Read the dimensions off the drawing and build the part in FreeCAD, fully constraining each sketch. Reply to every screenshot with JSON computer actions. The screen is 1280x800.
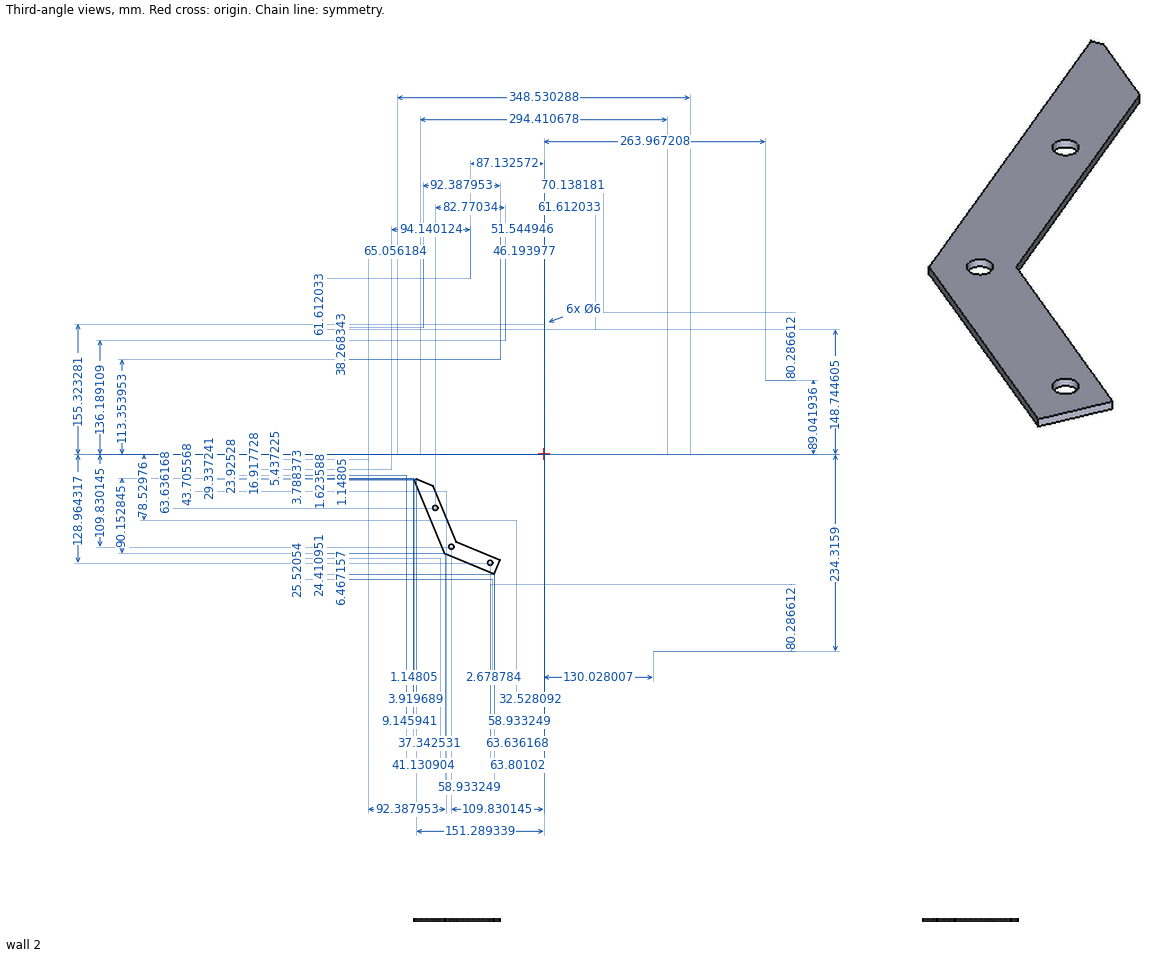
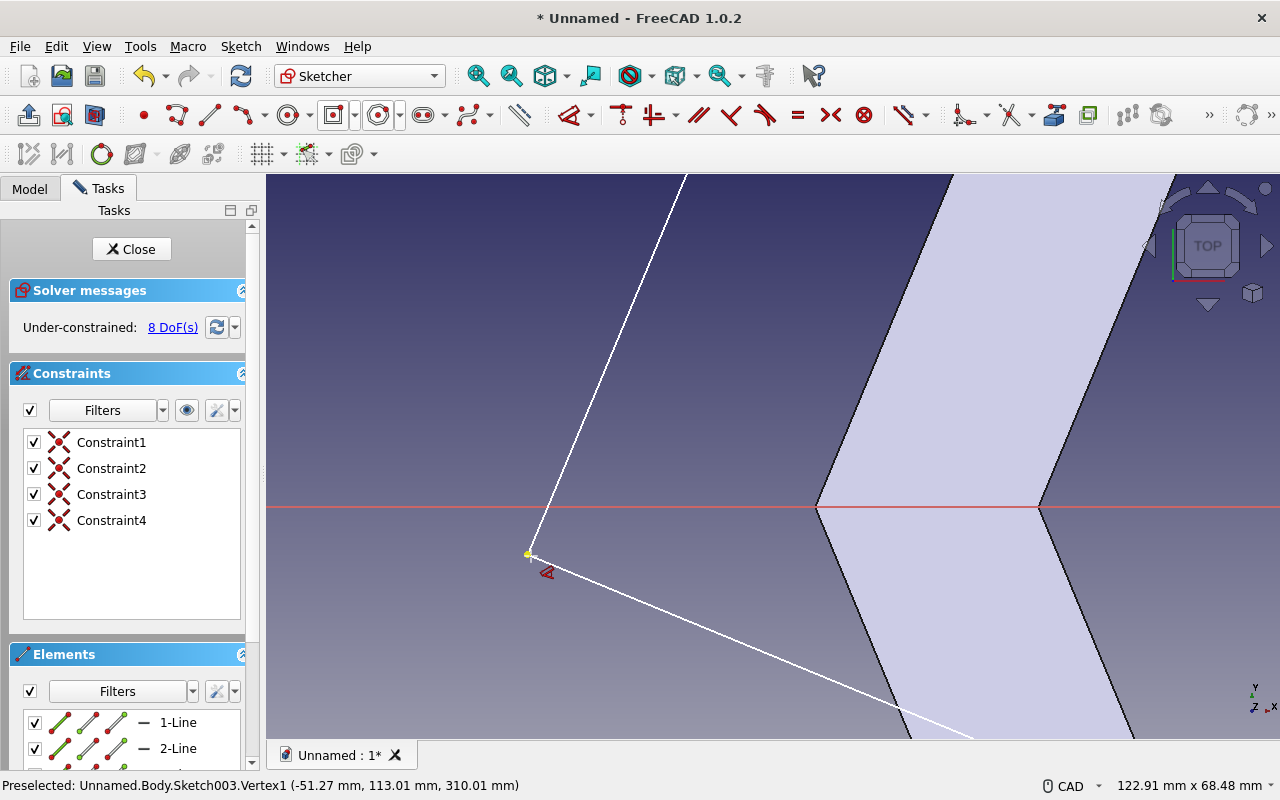
{"action": "left_click", "coordinate": [528, 555]}
{"action": "left_click", "coordinate": [494, 531]}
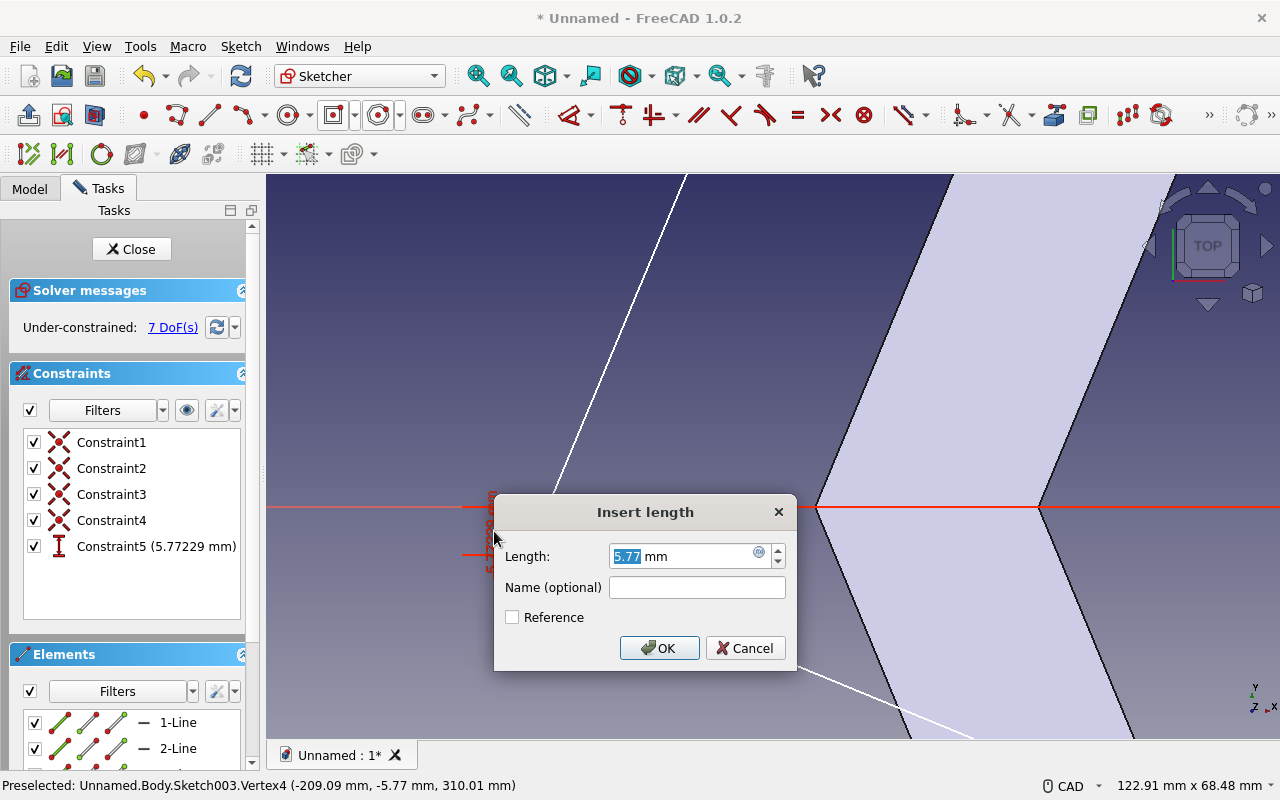
{"action": "type", "text": "5.437225"}
{"action": "key", "text": "Return"}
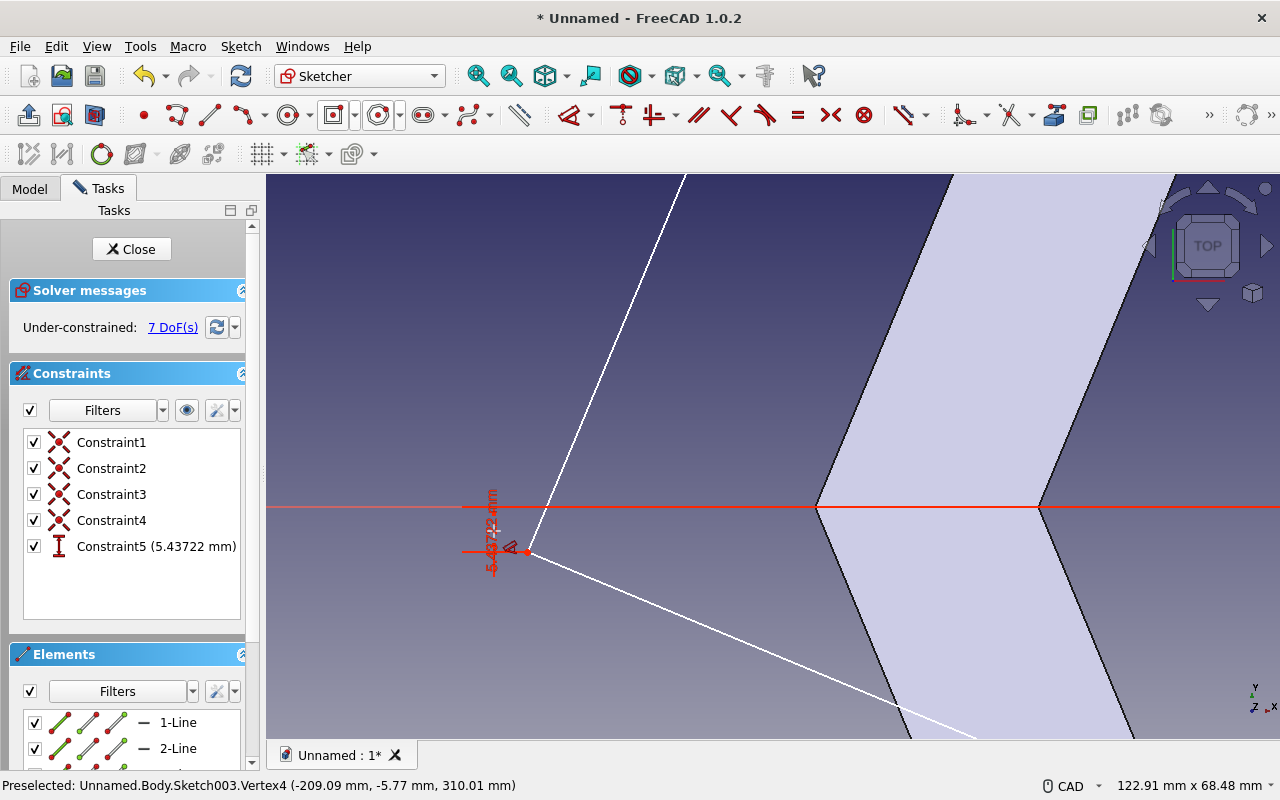
{"action": "scroll", "coordinate": [531, 556], "scroll_direction": "down", "scroll_amount": 8}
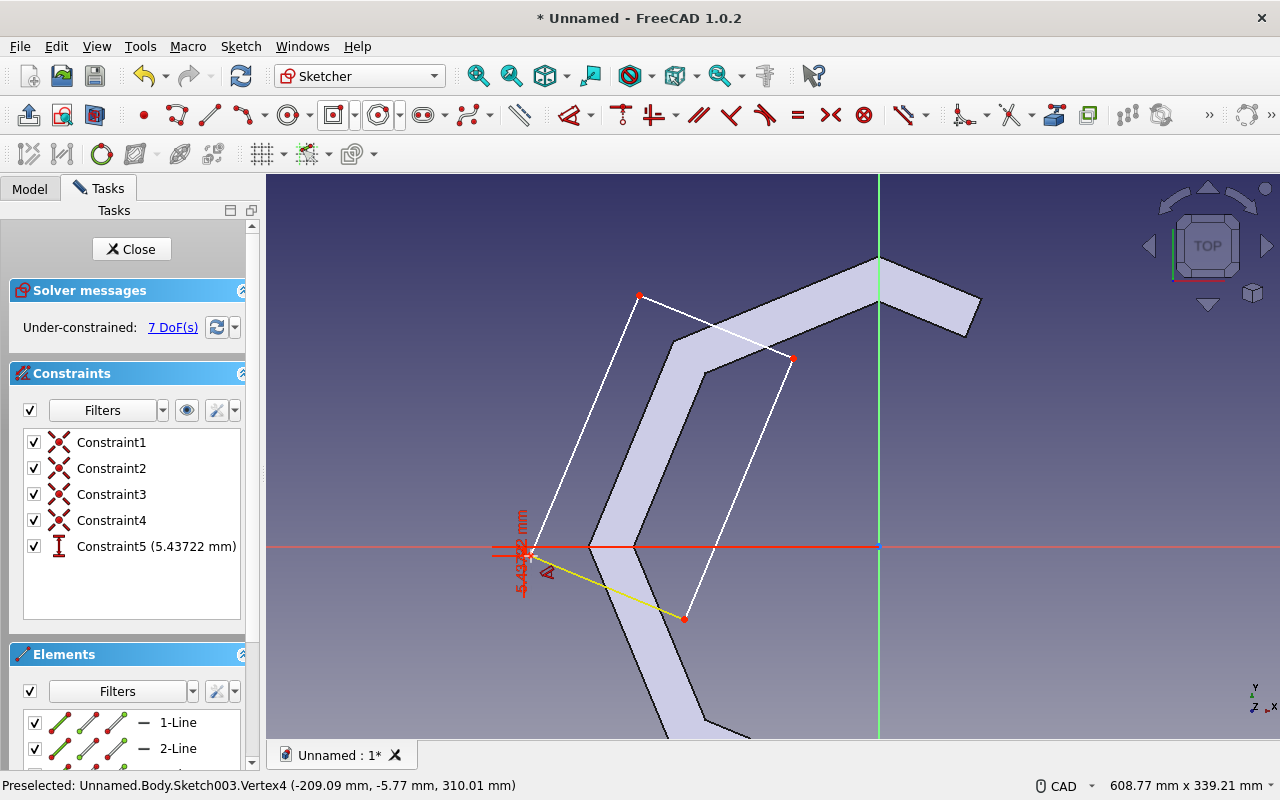
{"action": "left_click", "coordinate": [793, 358]}
{"action": "left_click", "coordinate": [836, 324]}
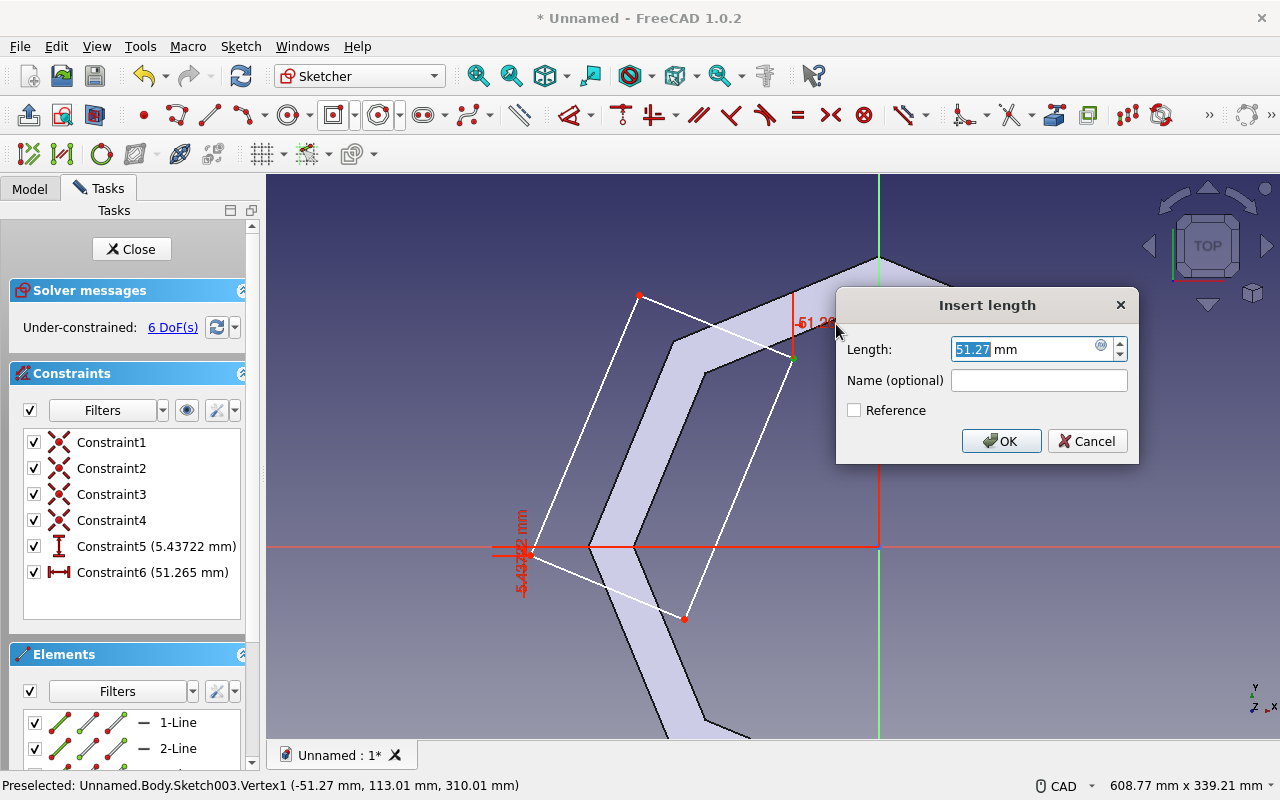
{"action": "type", "text": "51.544946"}
{"action": "key", "text": "Return"}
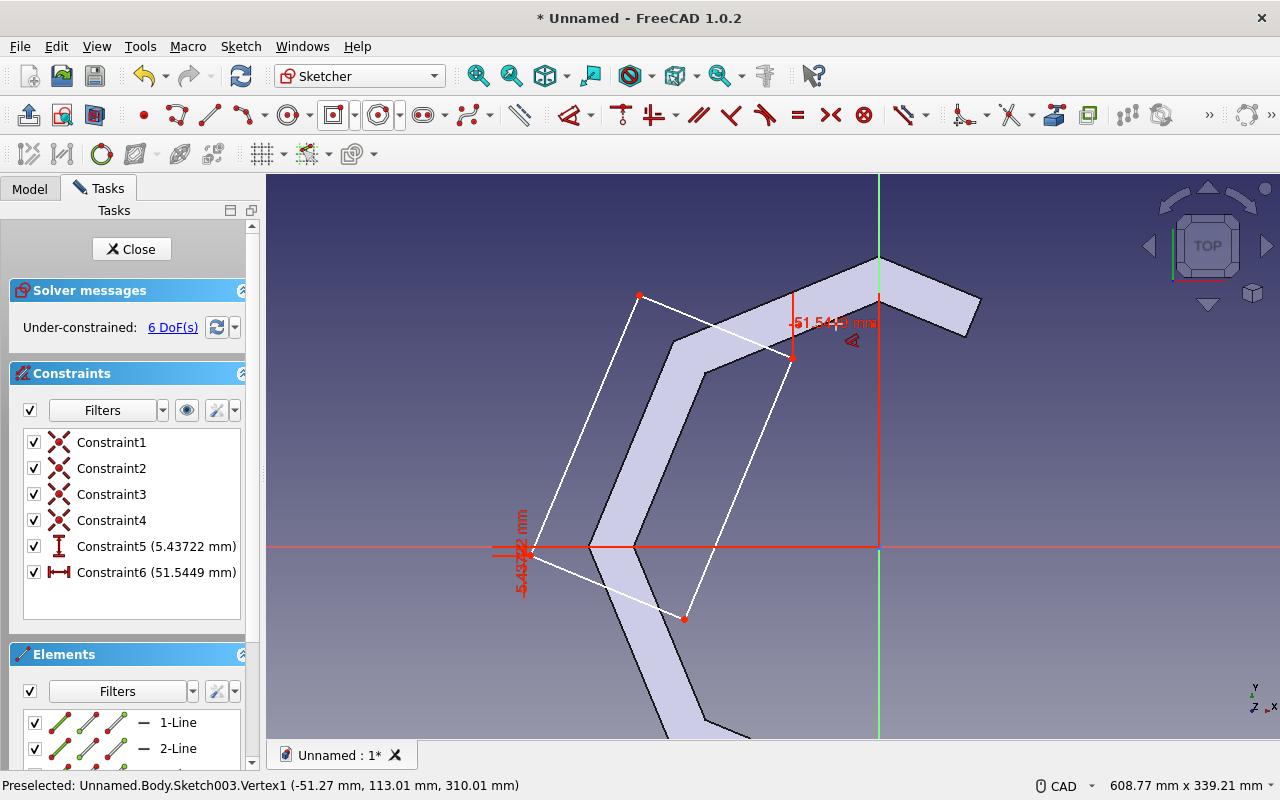
{"action": "left_click", "coordinate": [685, 620]}
{"action": "left_click", "coordinate": [913, 583]}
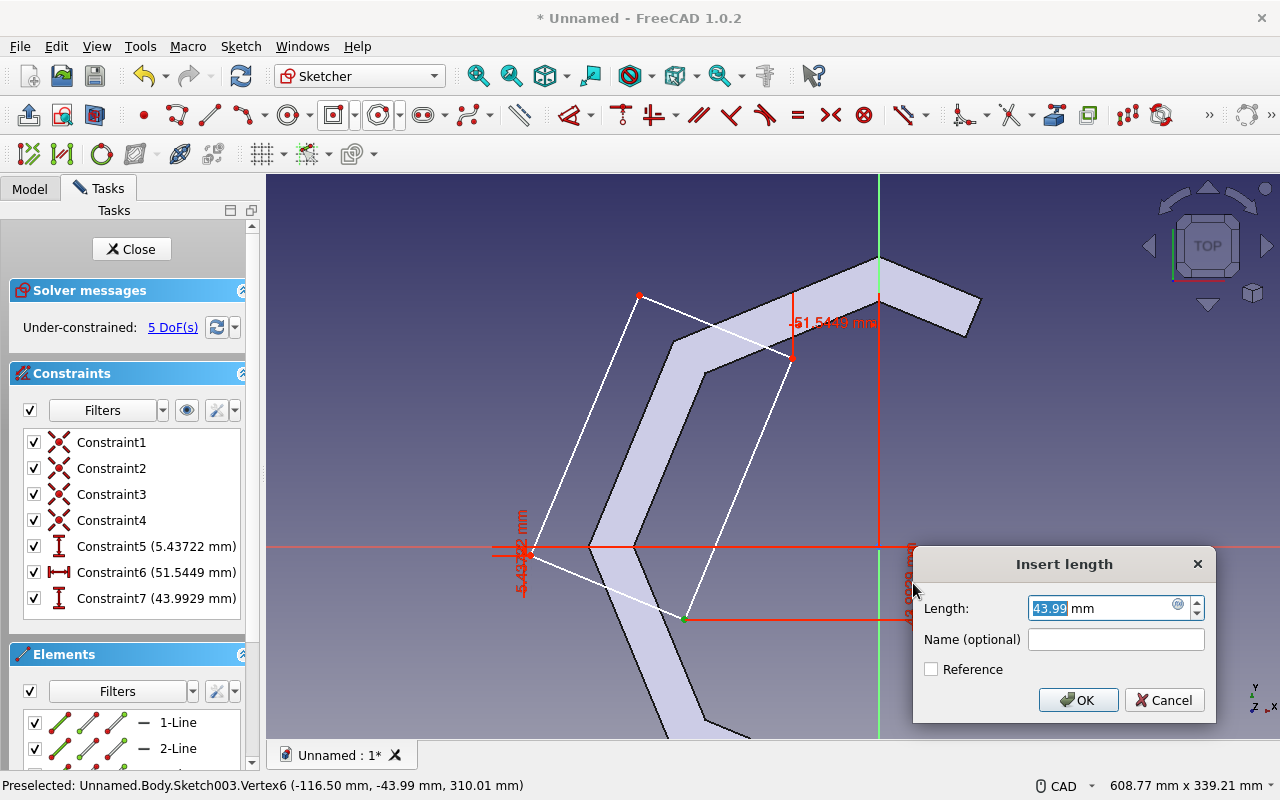
{"action": "type", "text": "43.705568"}
{"action": "key", "text": "Return"}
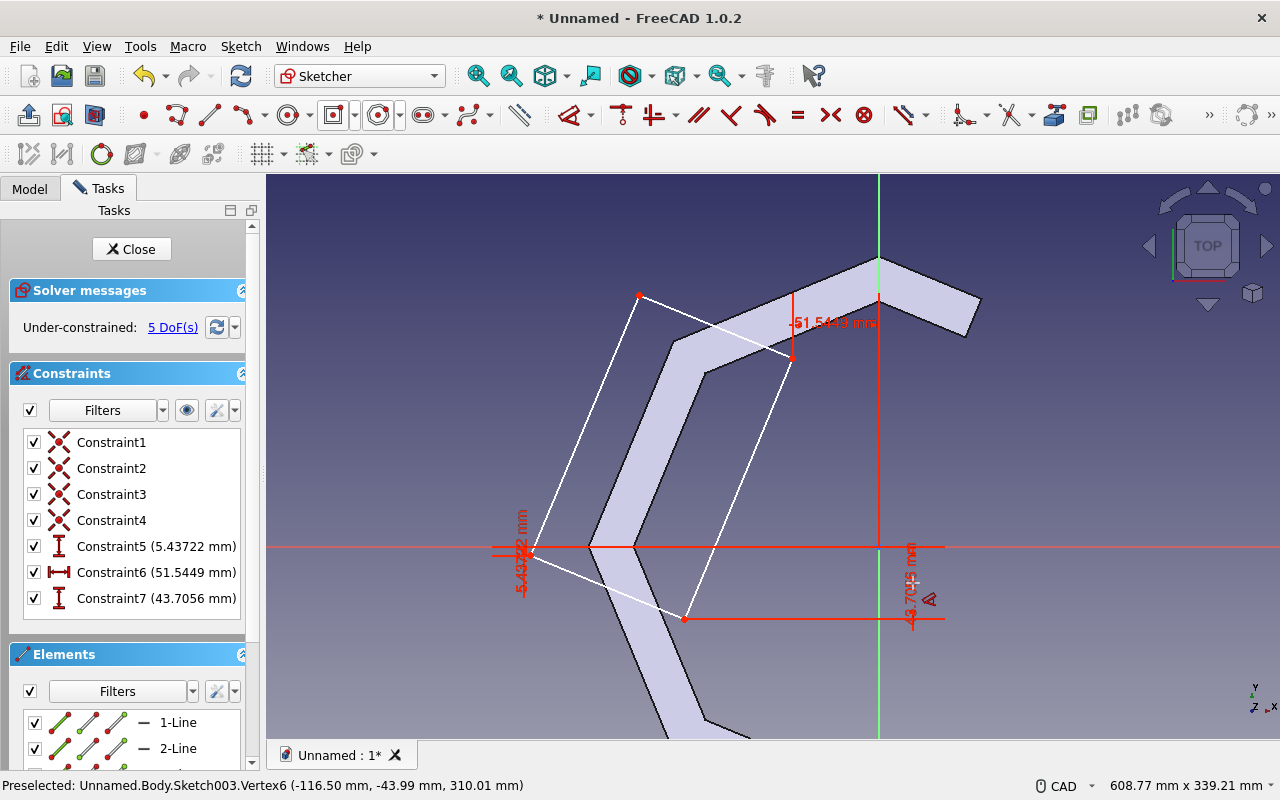
{"action": "left_click", "coordinate": [747, 340]}
{"action": "left_click", "coordinate": [716, 261]}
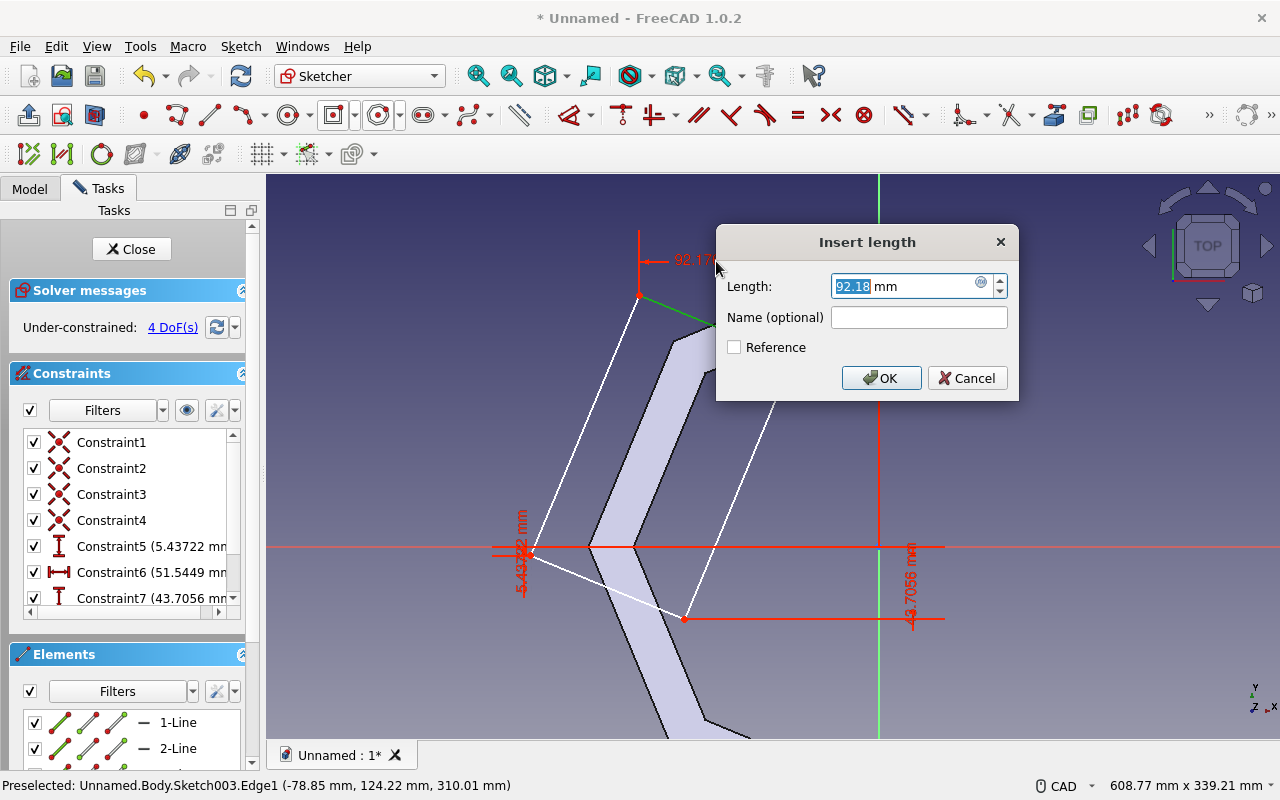
{"action": "type", "text": "92.387953"}
{"action": "key", "text": "Return"}